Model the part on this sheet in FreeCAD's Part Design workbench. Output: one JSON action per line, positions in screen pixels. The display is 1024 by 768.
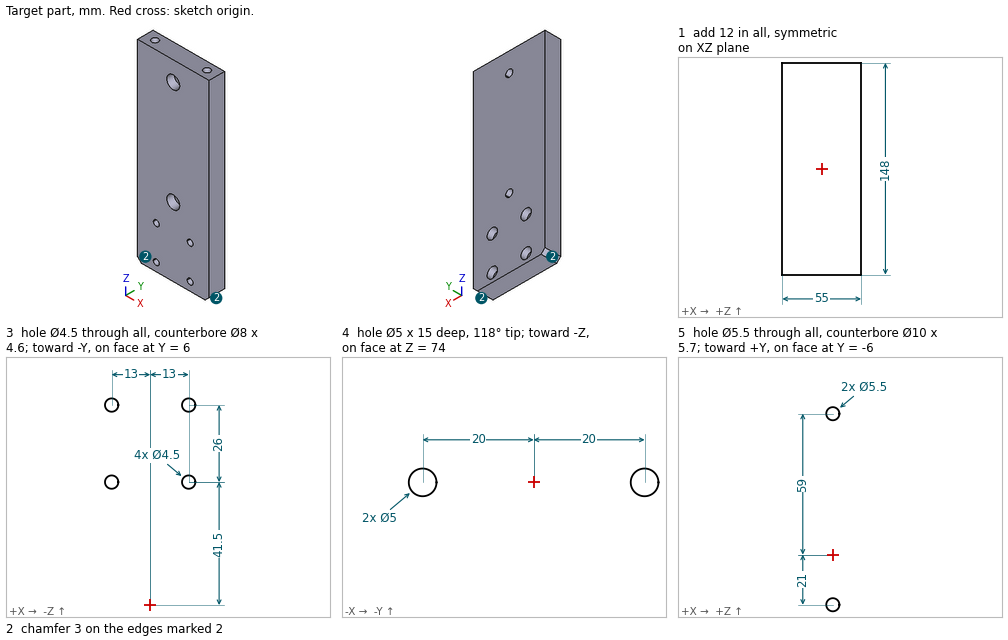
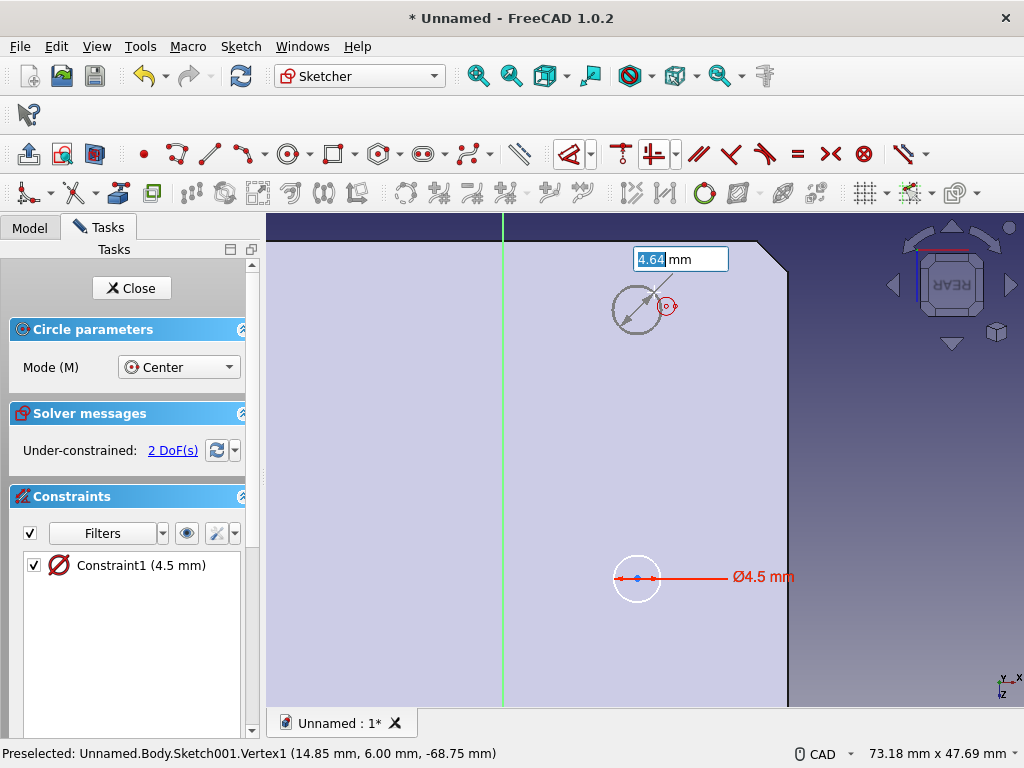
{"action": "type", "text": "4.5"}
{"action": "key", "text": "Return"}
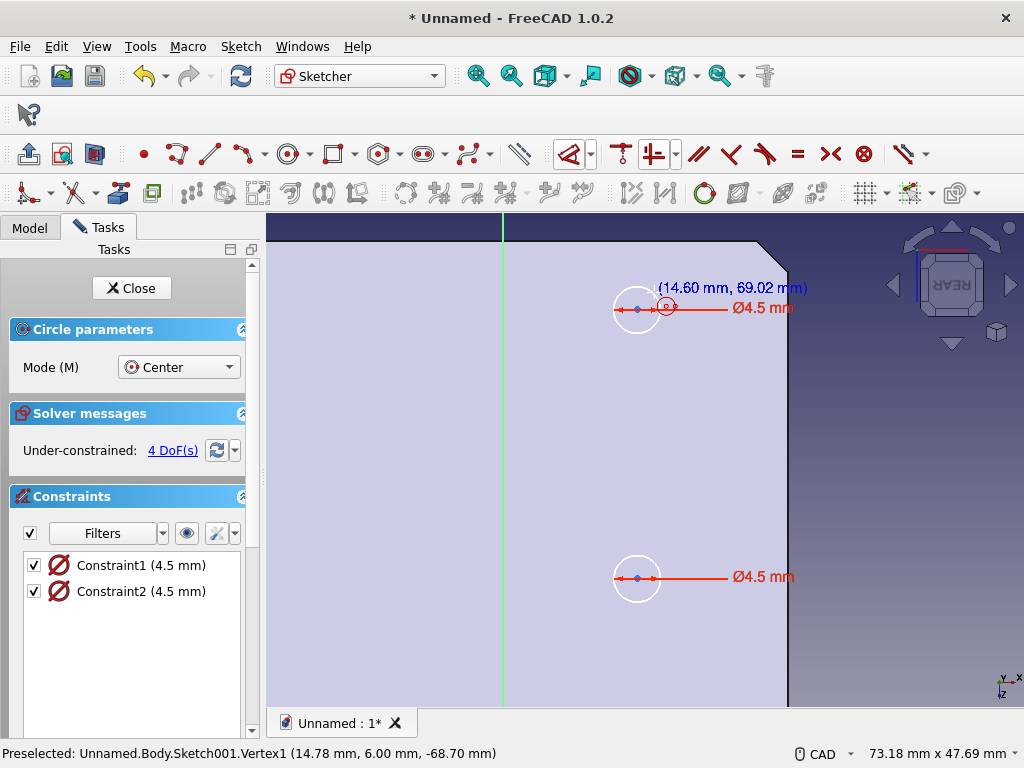
{"action": "left_click", "coordinate": [368, 309]}
{"action": "mouse_move", "coordinate": [385, 292]}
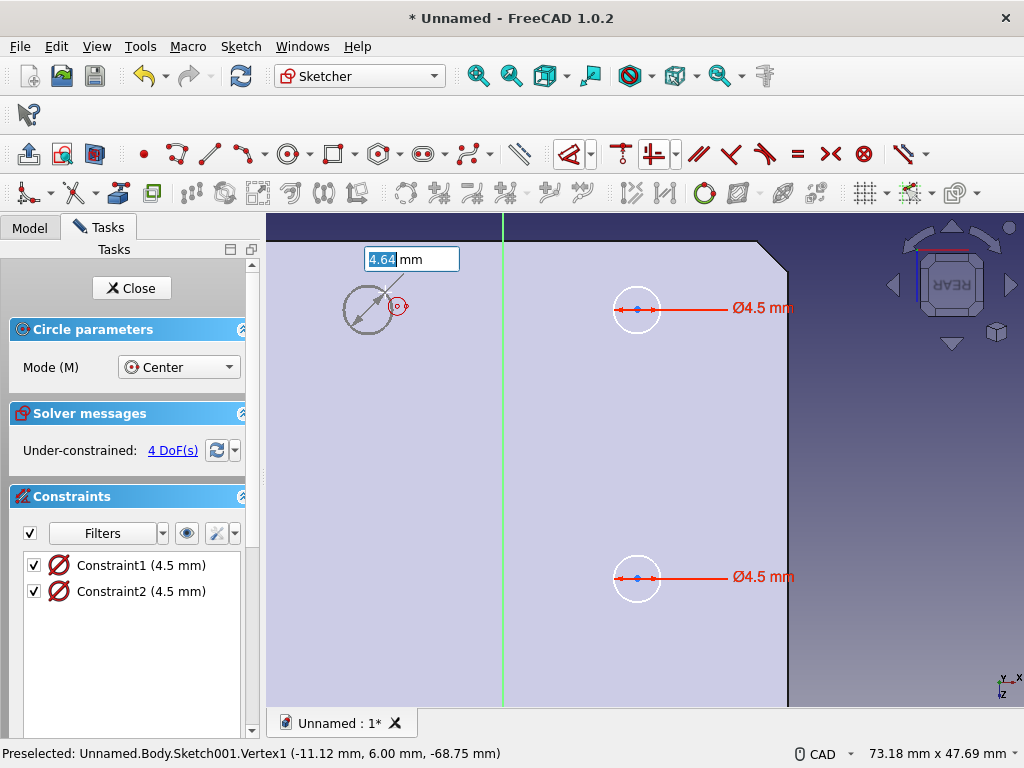
{"action": "type", "text": "4.5"}
{"action": "key", "text": "Return"}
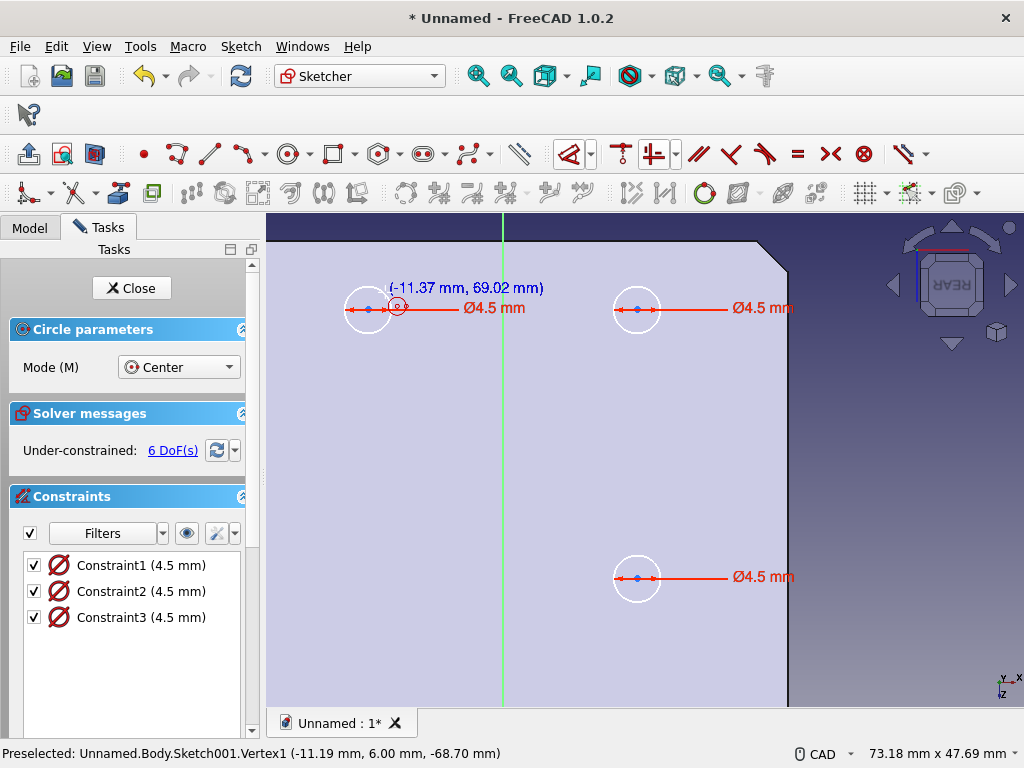
{"action": "left_click", "coordinate": [368, 578]}
{"action": "mouse_move", "coordinate": [385, 562]}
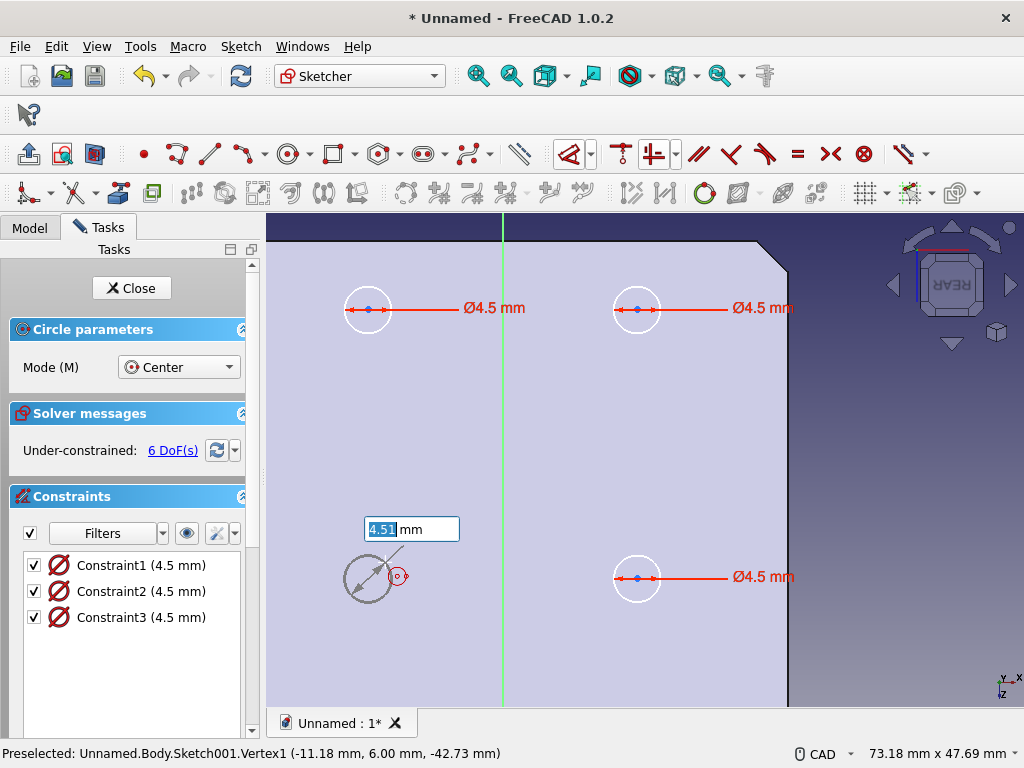
{"action": "type", "text": "4.5"}
{"action": "key", "text": "Return"}
{"action": "key", "text": "Escape"}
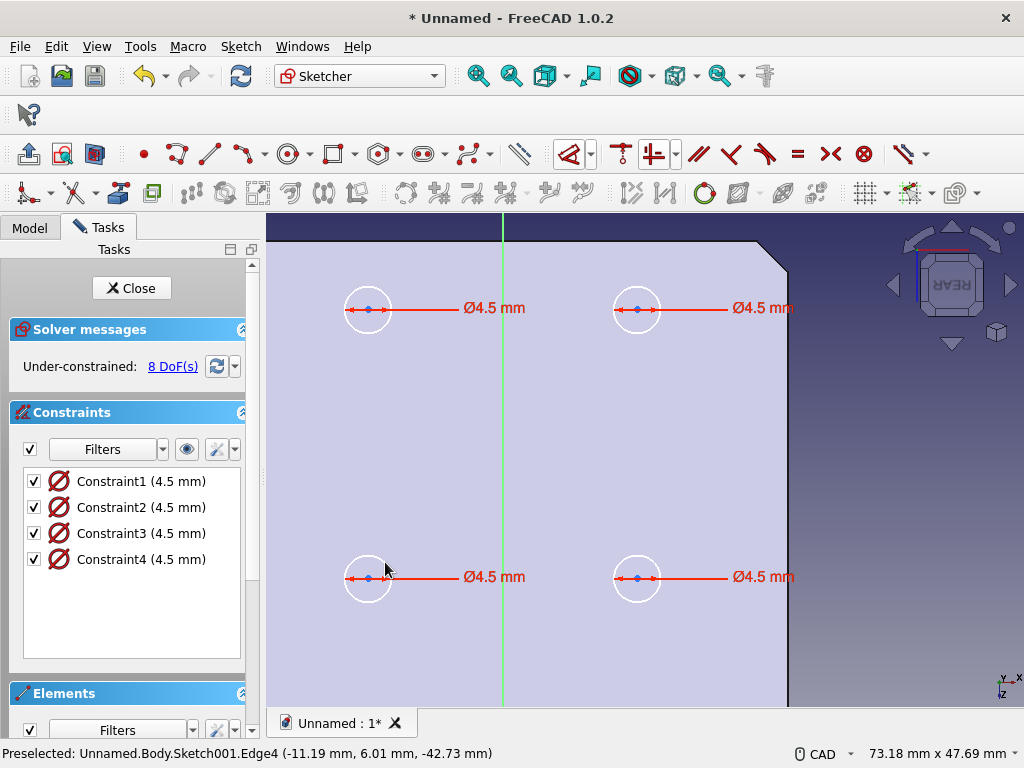
{"action": "left_click", "coordinate": [637, 579]}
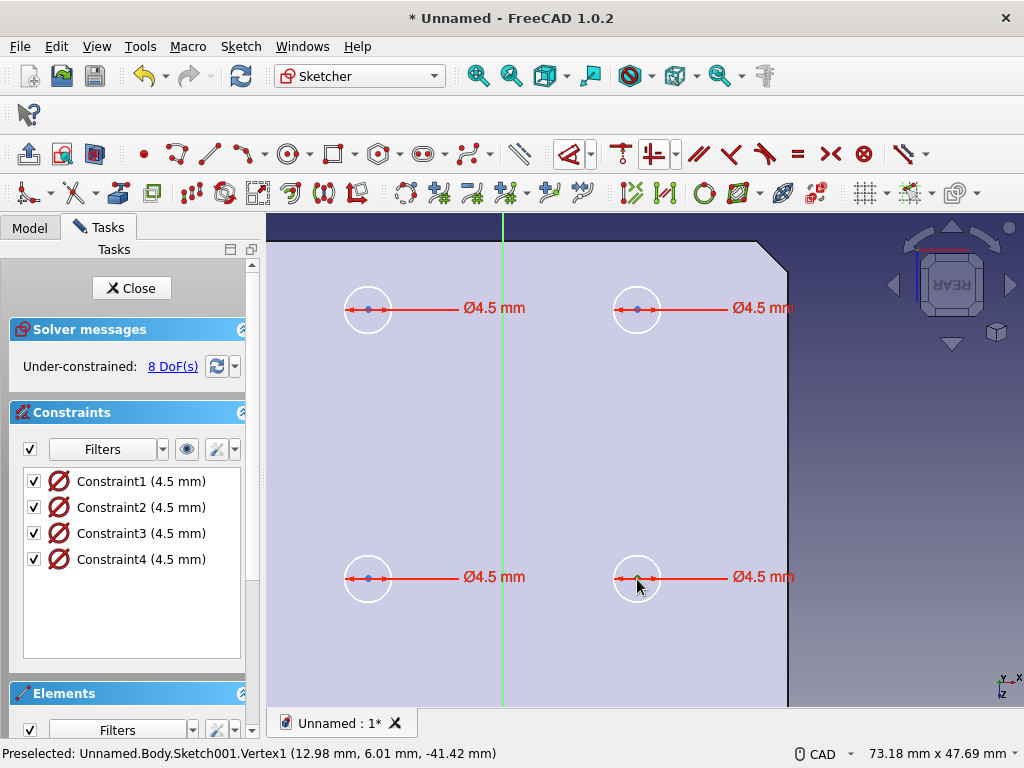
{"action": "left_click", "coordinate": [637, 310]}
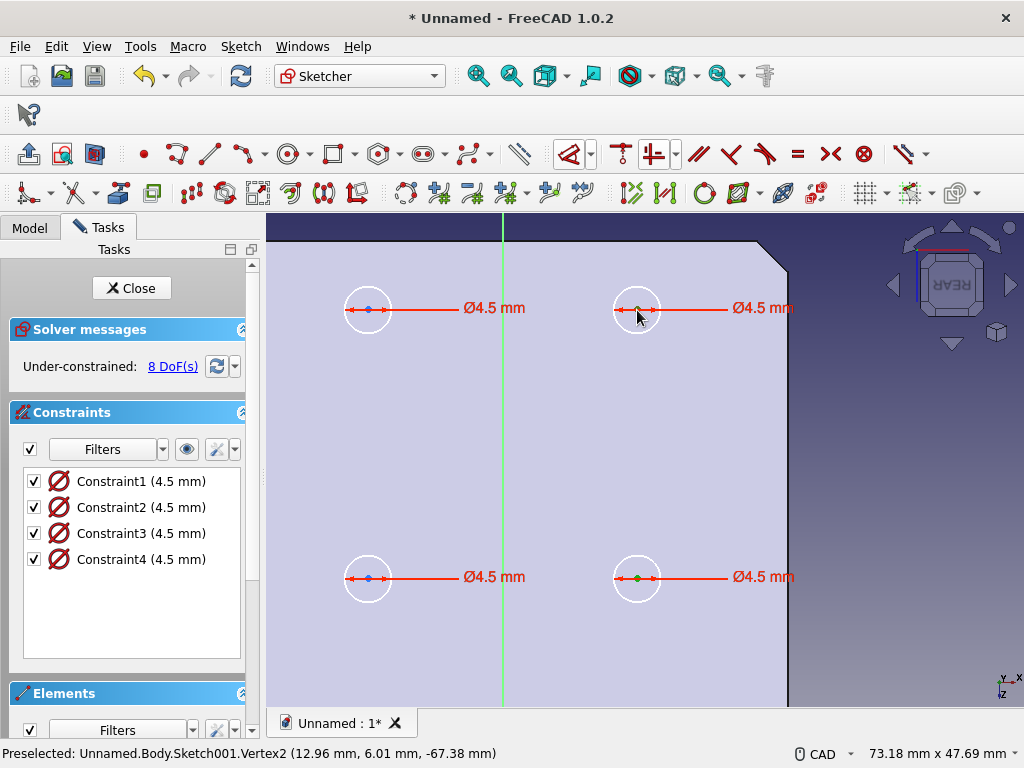
{"action": "left_click", "coordinate": [676, 154]}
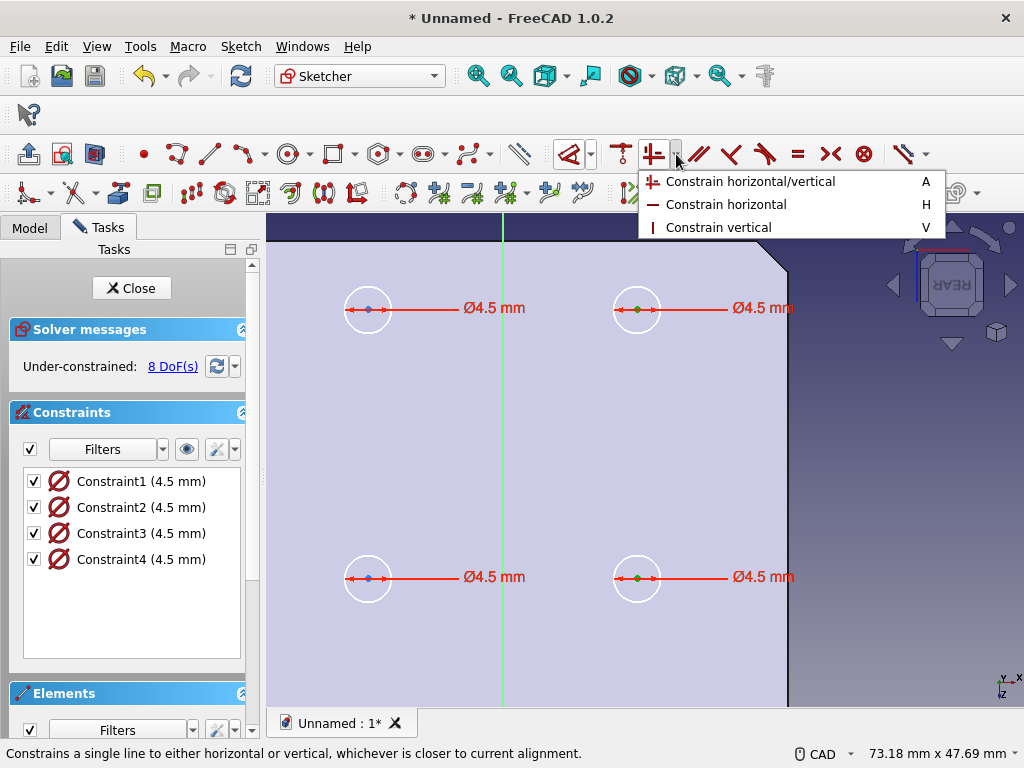
{"action": "left_click", "coordinate": [792, 228]}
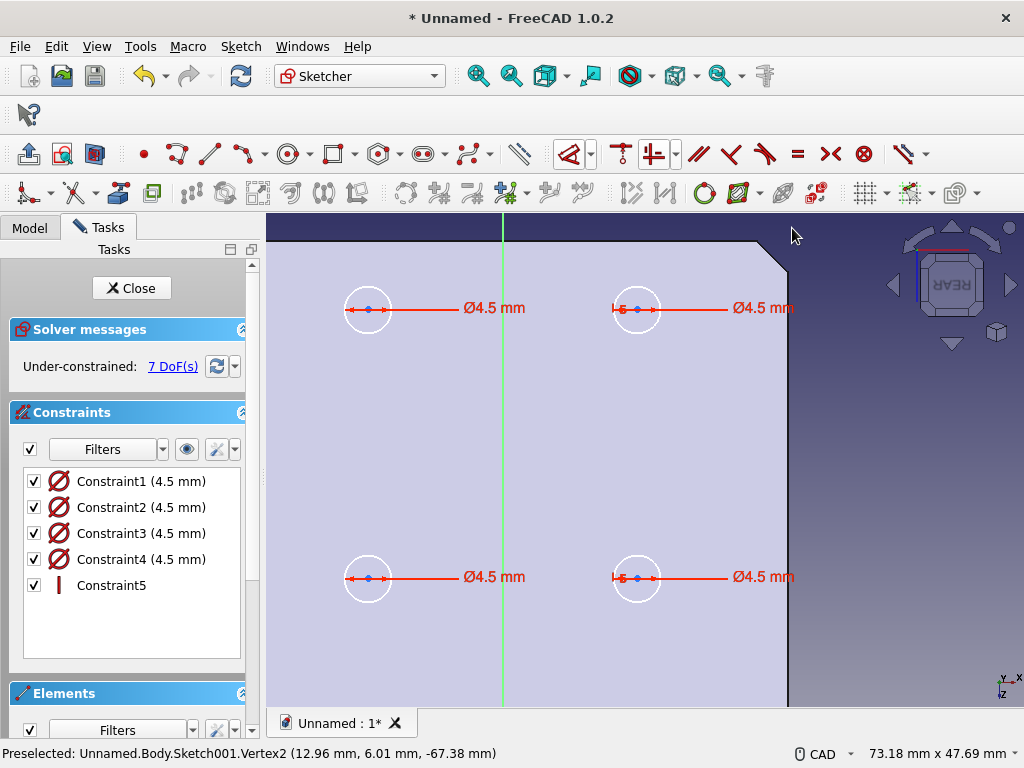
{"action": "left_click", "coordinate": [637, 310]}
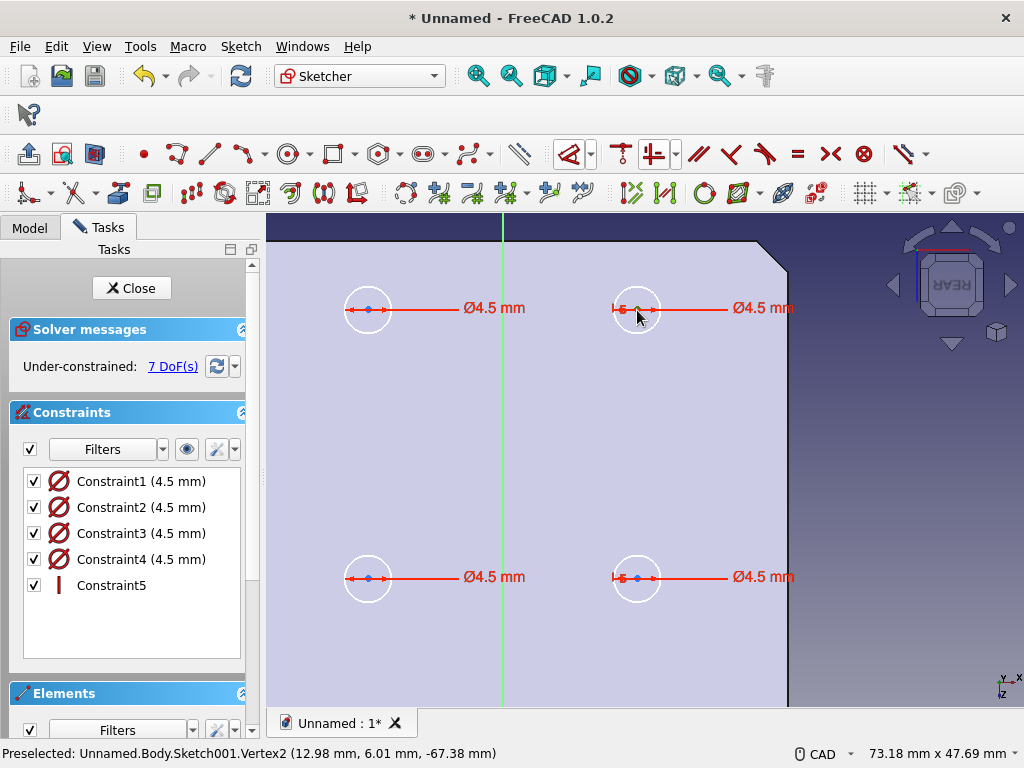
{"action": "left_click", "coordinate": [368, 310]}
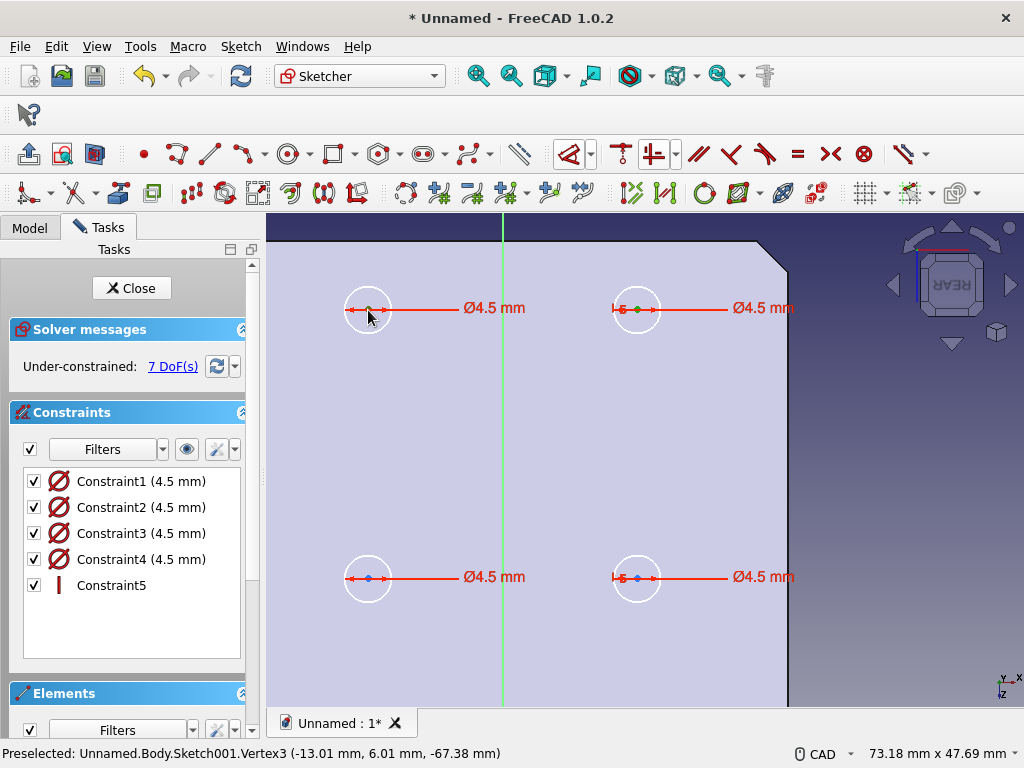
{"action": "key", "text": "h"}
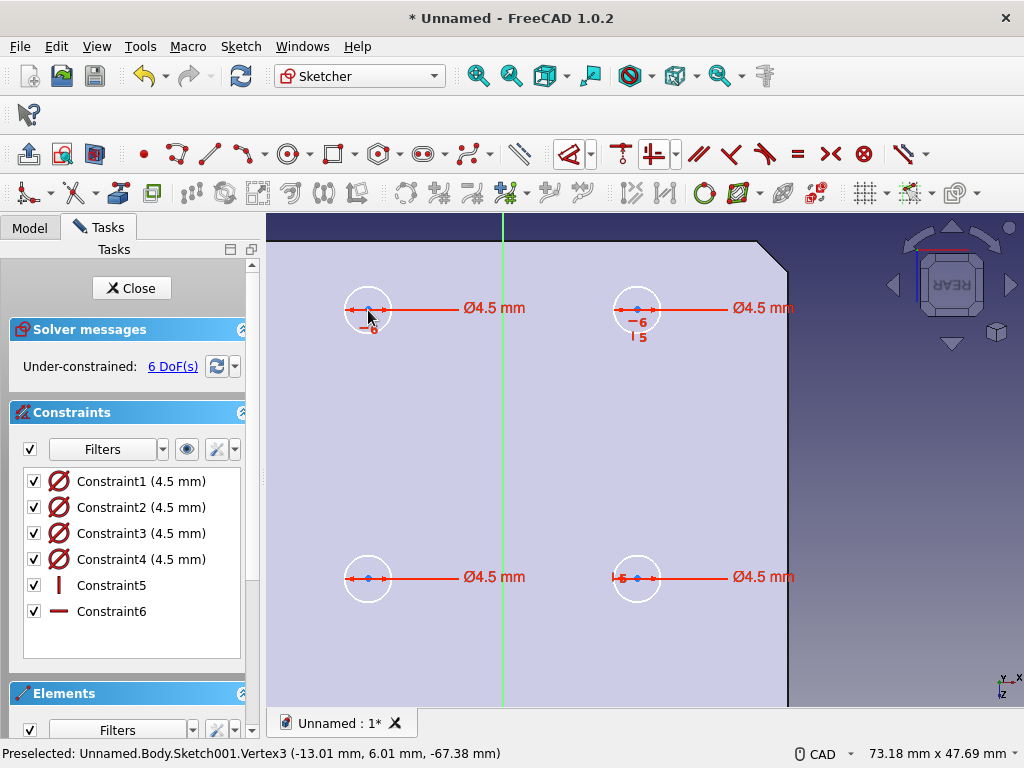
{"action": "left_click", "coordinate": [368, 310]}